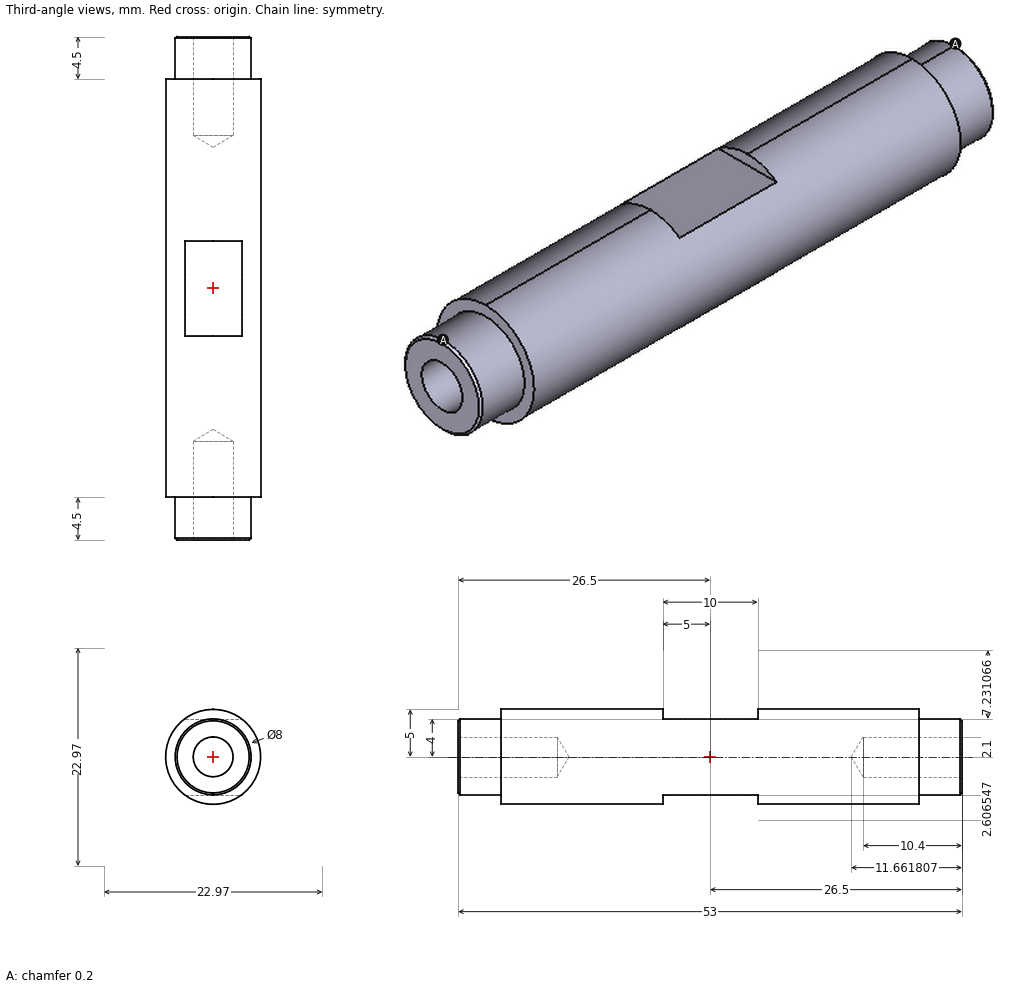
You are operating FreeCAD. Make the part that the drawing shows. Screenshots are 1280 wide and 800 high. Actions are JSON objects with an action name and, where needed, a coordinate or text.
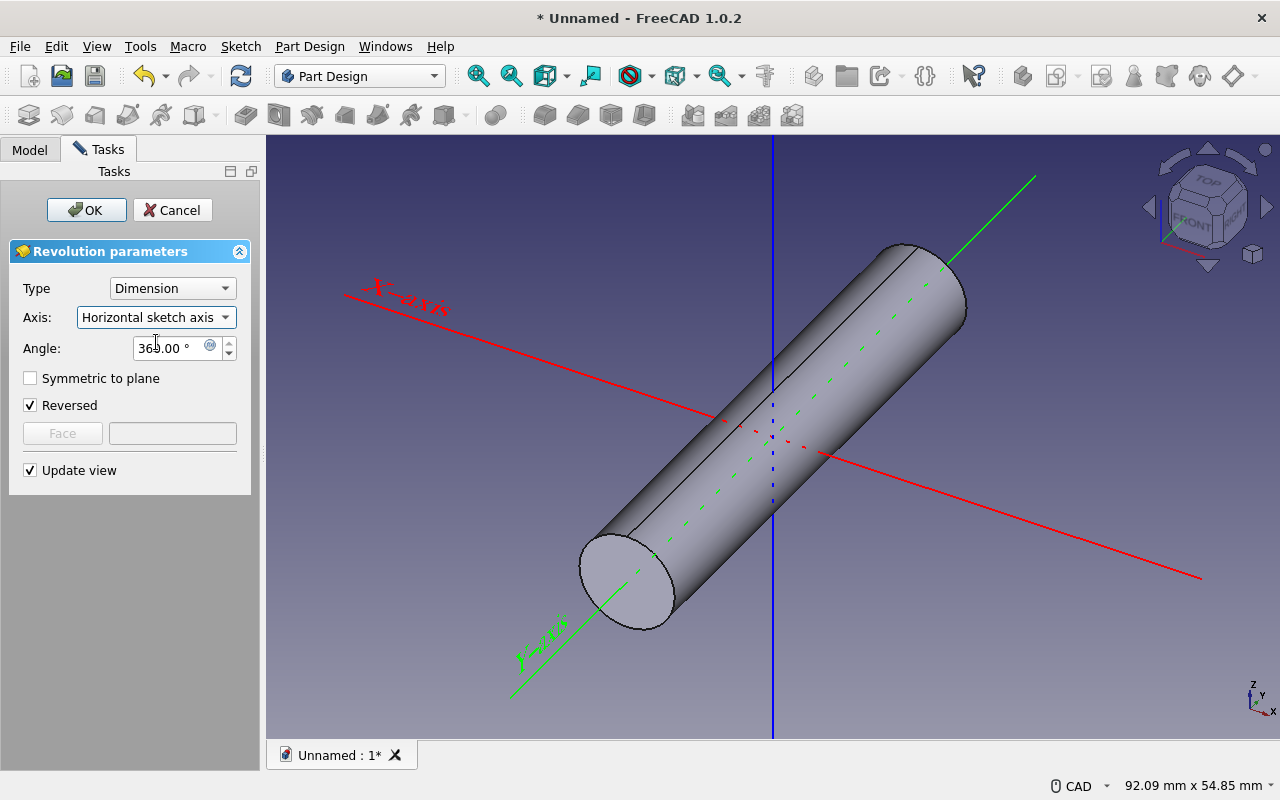
{"action": "left_click", "coordinate": [87, 210]}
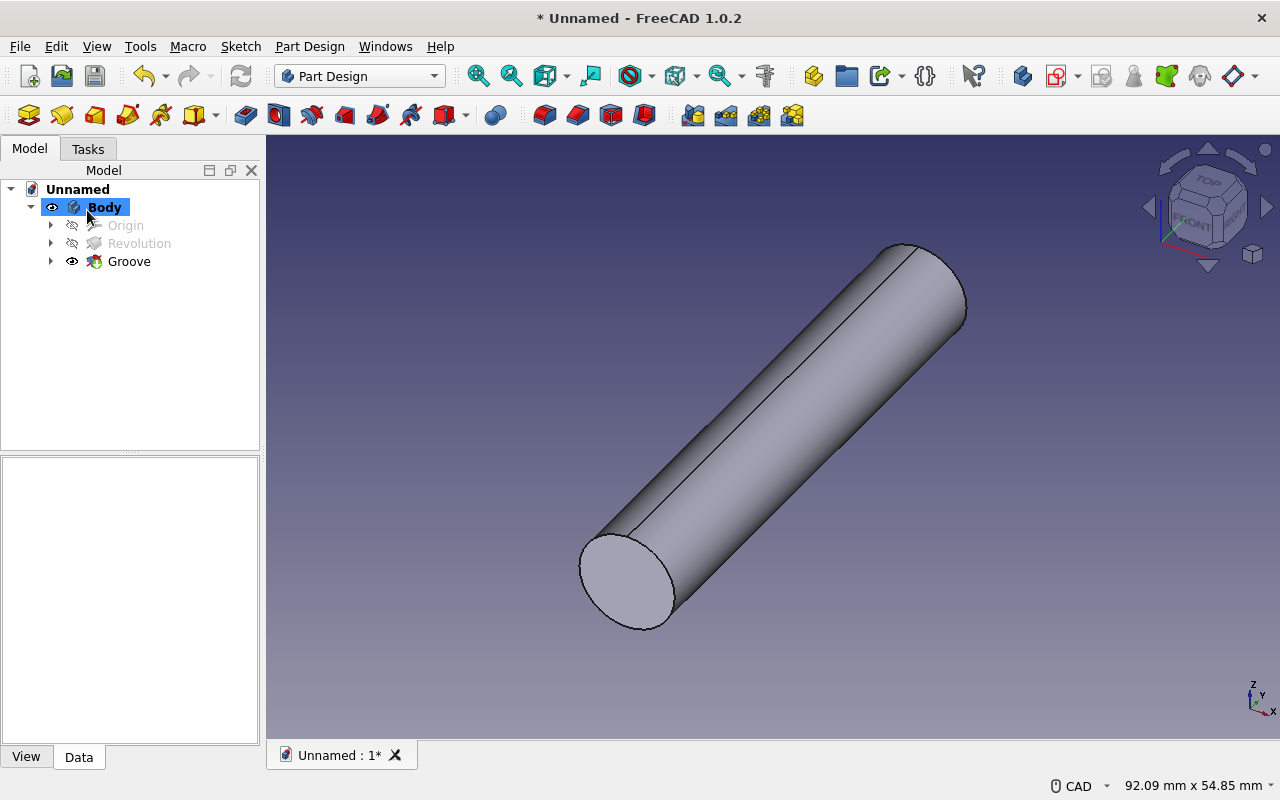
{"action": "left_click", "coordinate": [117, 261]}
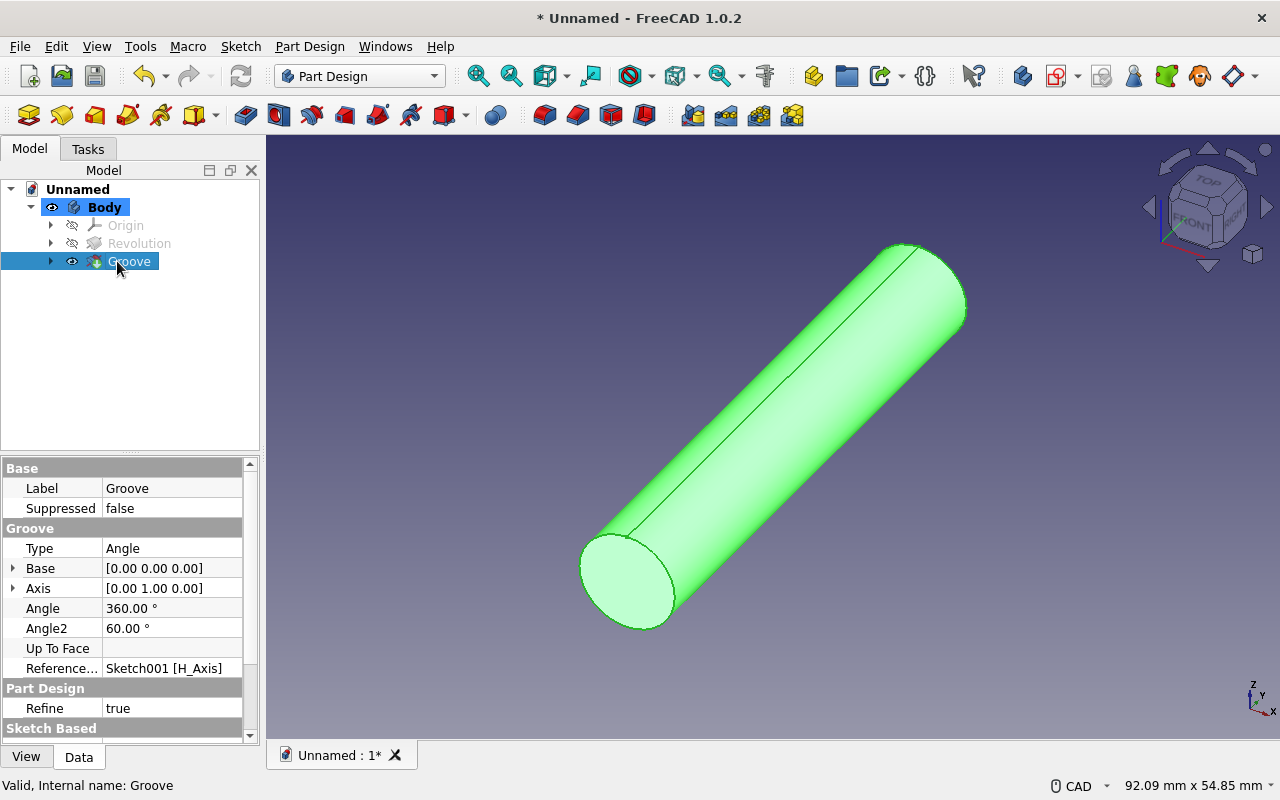
{"action": "left_click", "coordinate": [693, 116]}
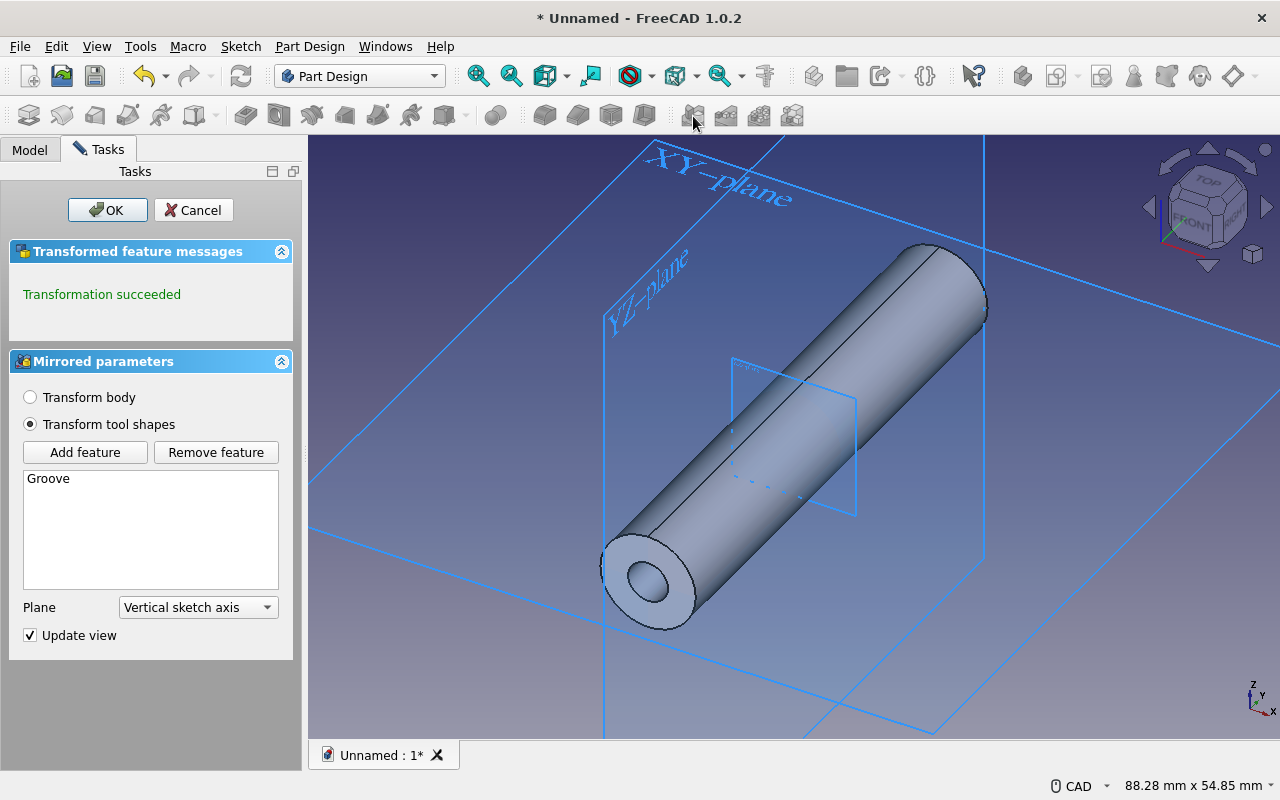
{"action": "left_click", "coordinate": [199, 608]}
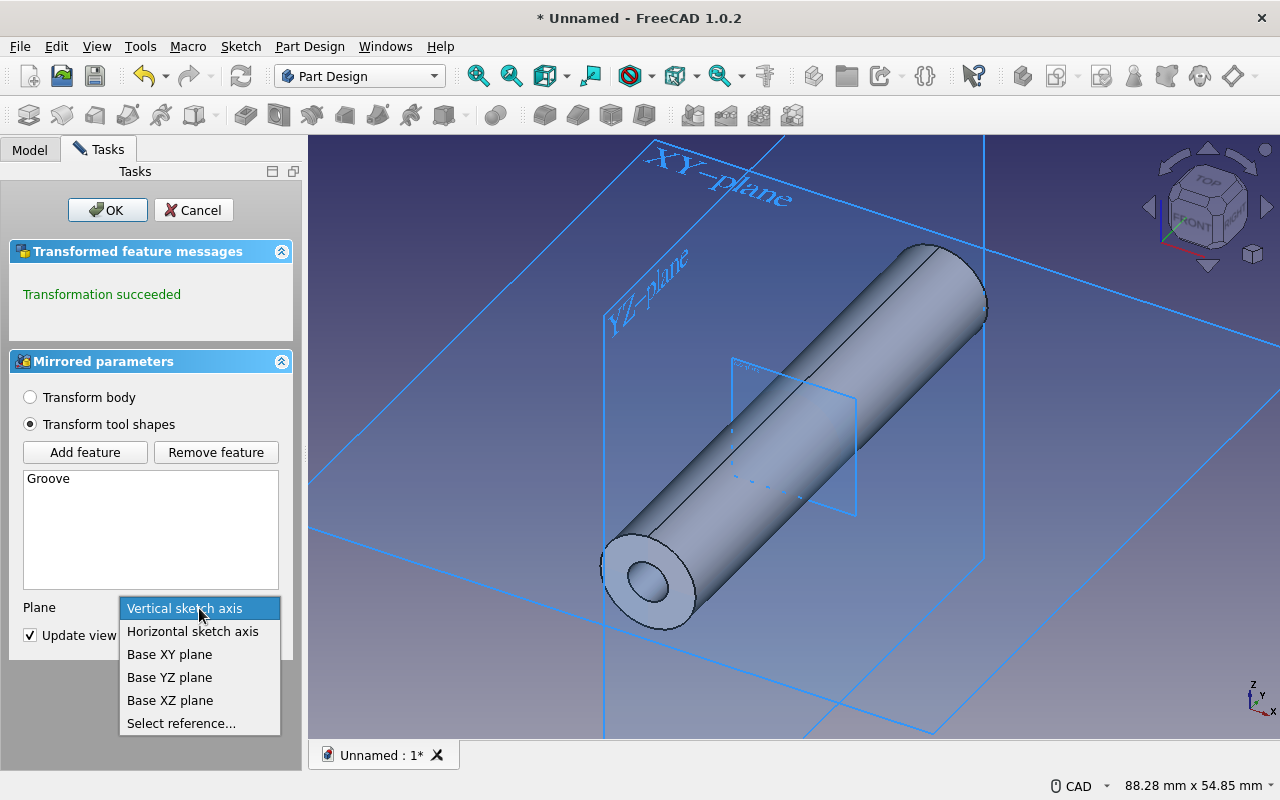
{"action": "left_click", "coordinate": [198, 700]}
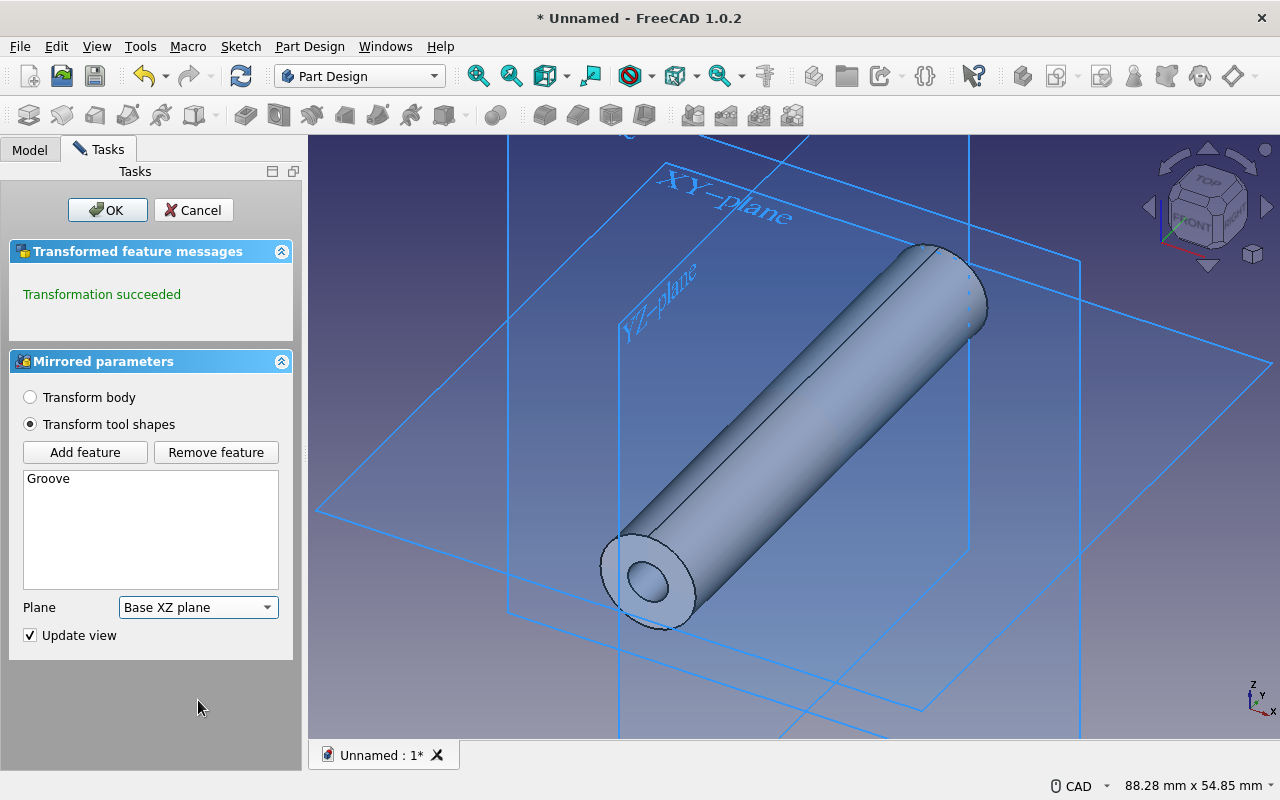
{"action": "left_click", "coordinate": [108, 210]}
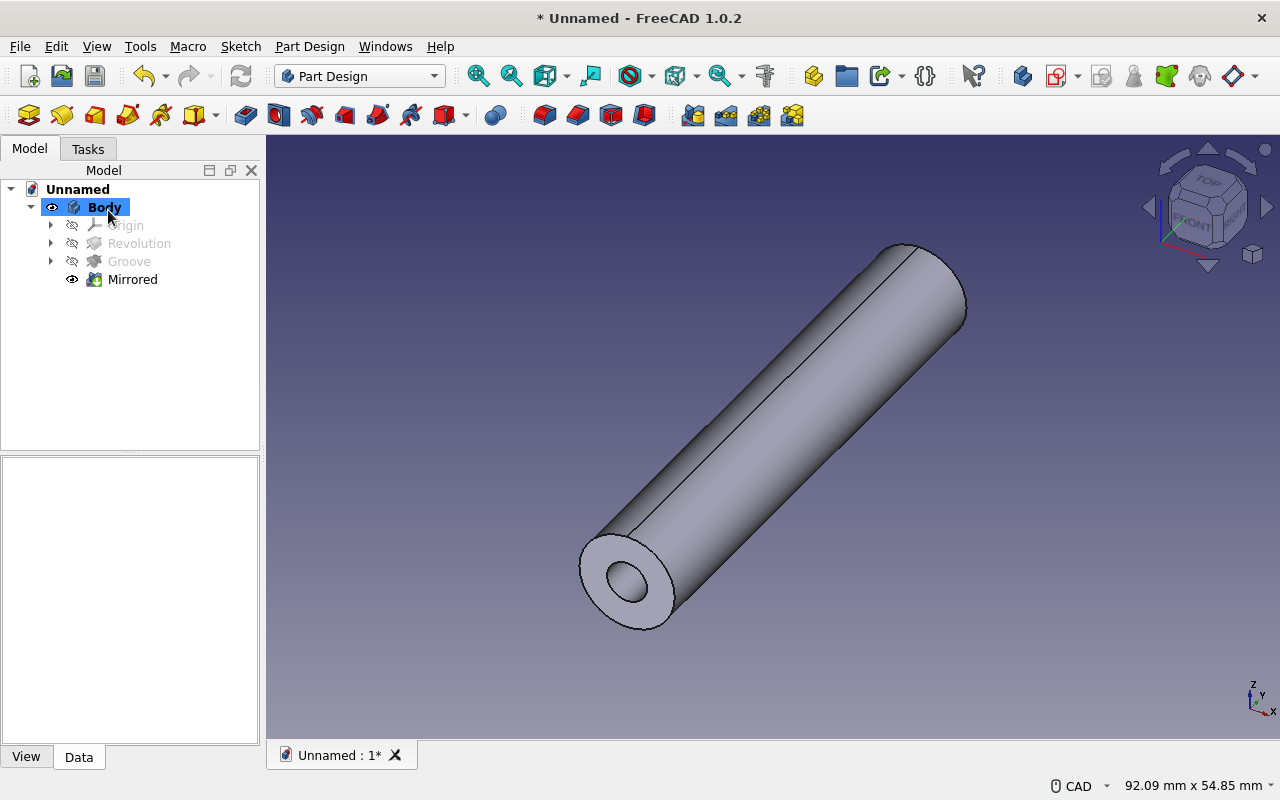
{"action": "left_click", "coordinate": [641, 560]}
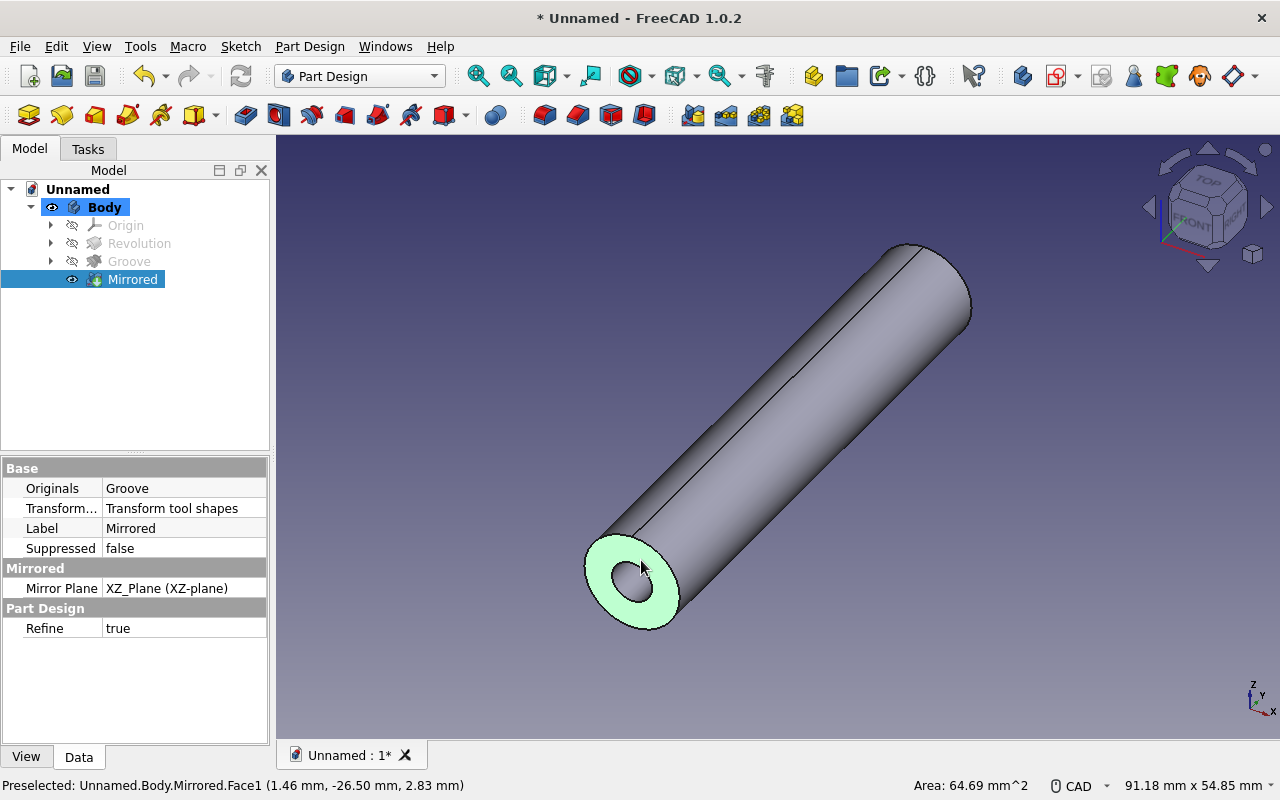
{"action": "left_click", "coordinate": [1056, 76]}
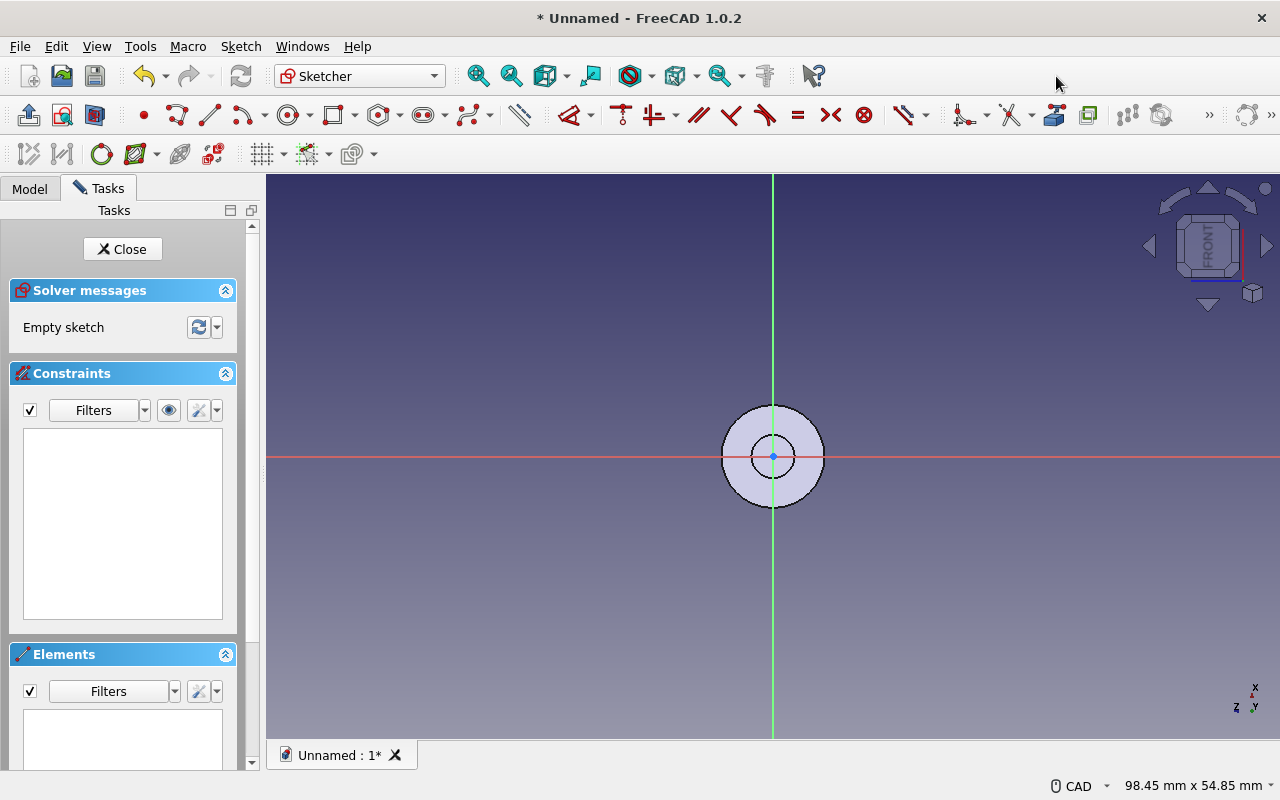
{"action": "scroll", "coordinate": [912, 457], "scroll_direction": "up", "scroll_amount": 2}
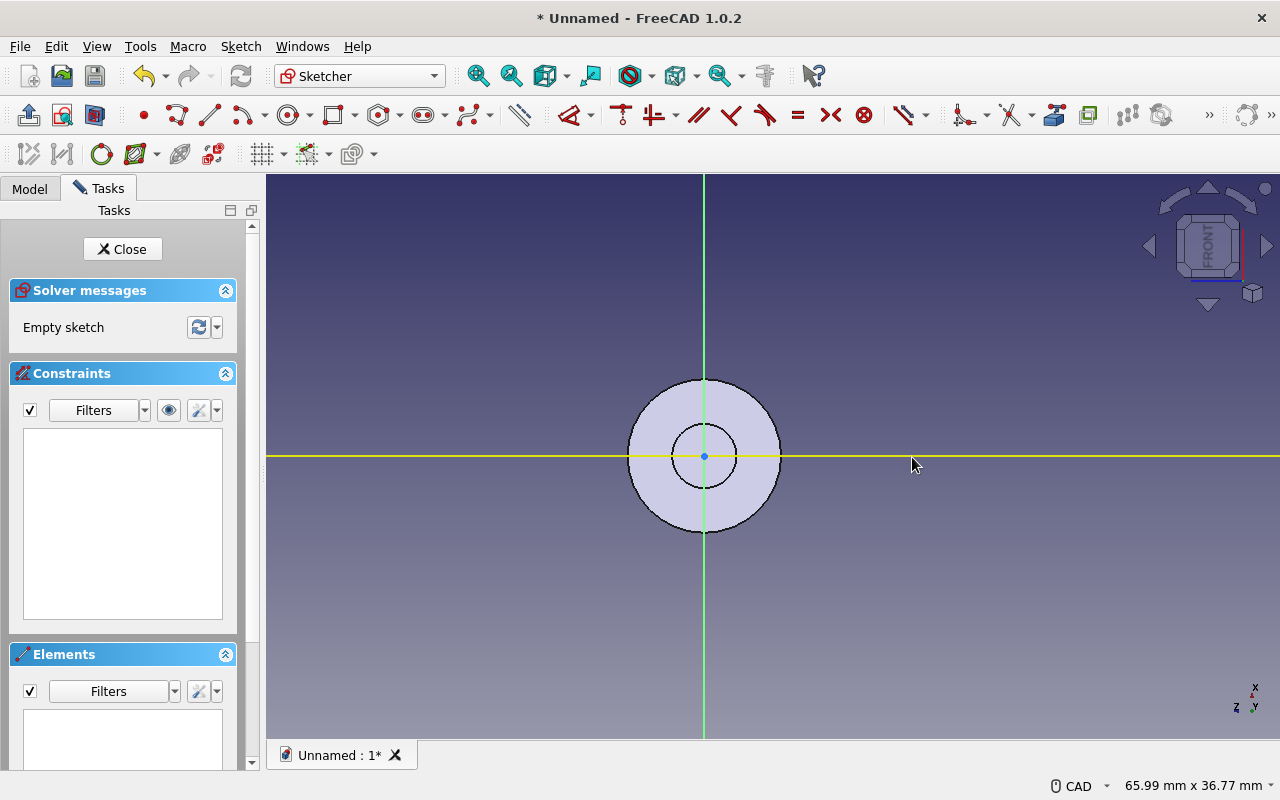
{"action": "key", "text": "g v"}